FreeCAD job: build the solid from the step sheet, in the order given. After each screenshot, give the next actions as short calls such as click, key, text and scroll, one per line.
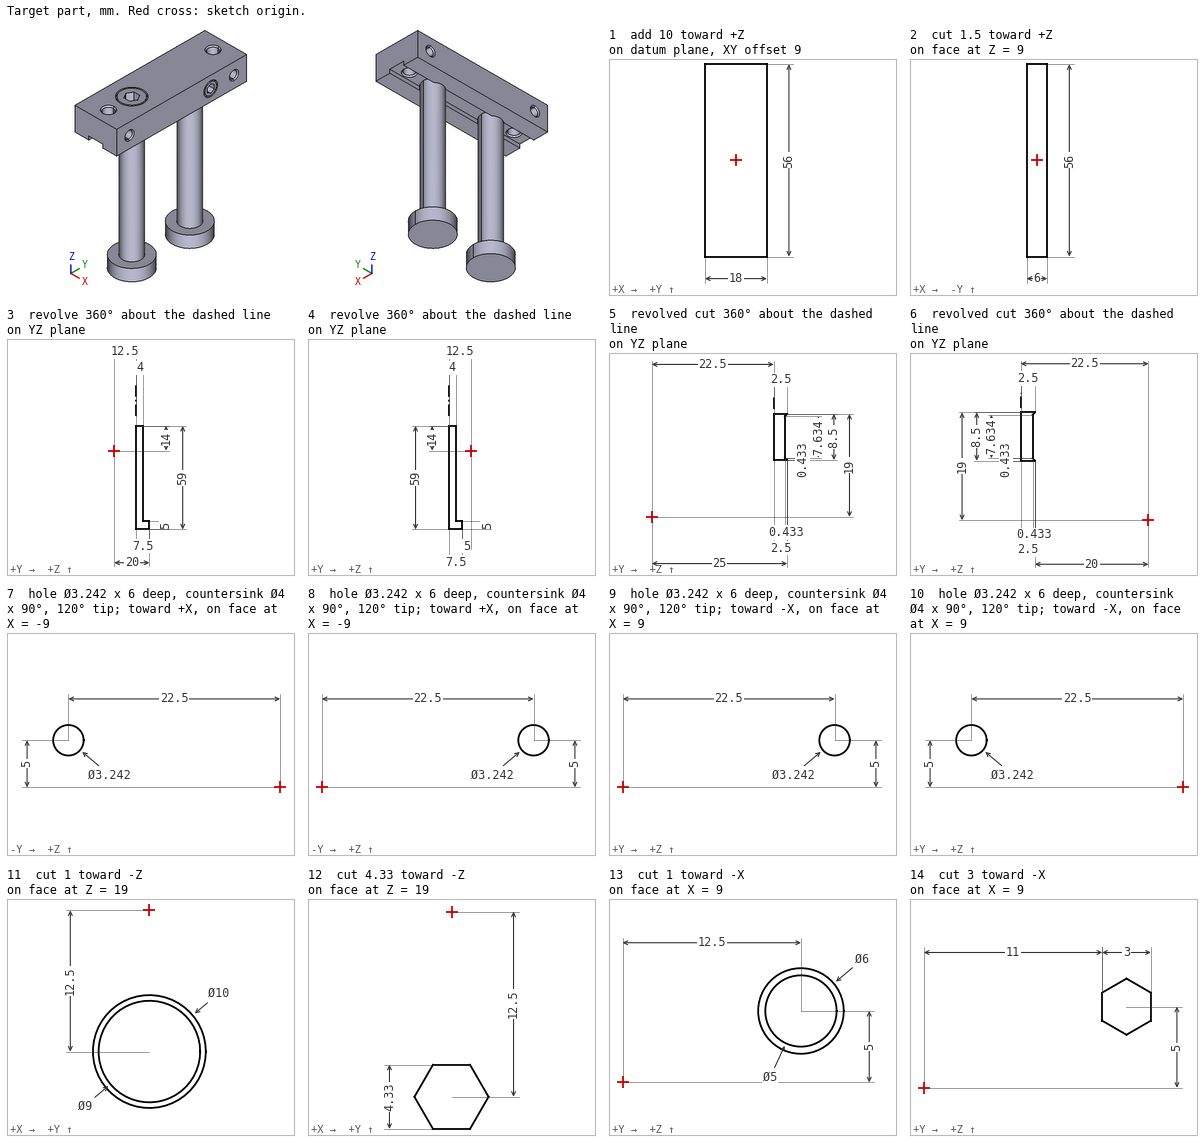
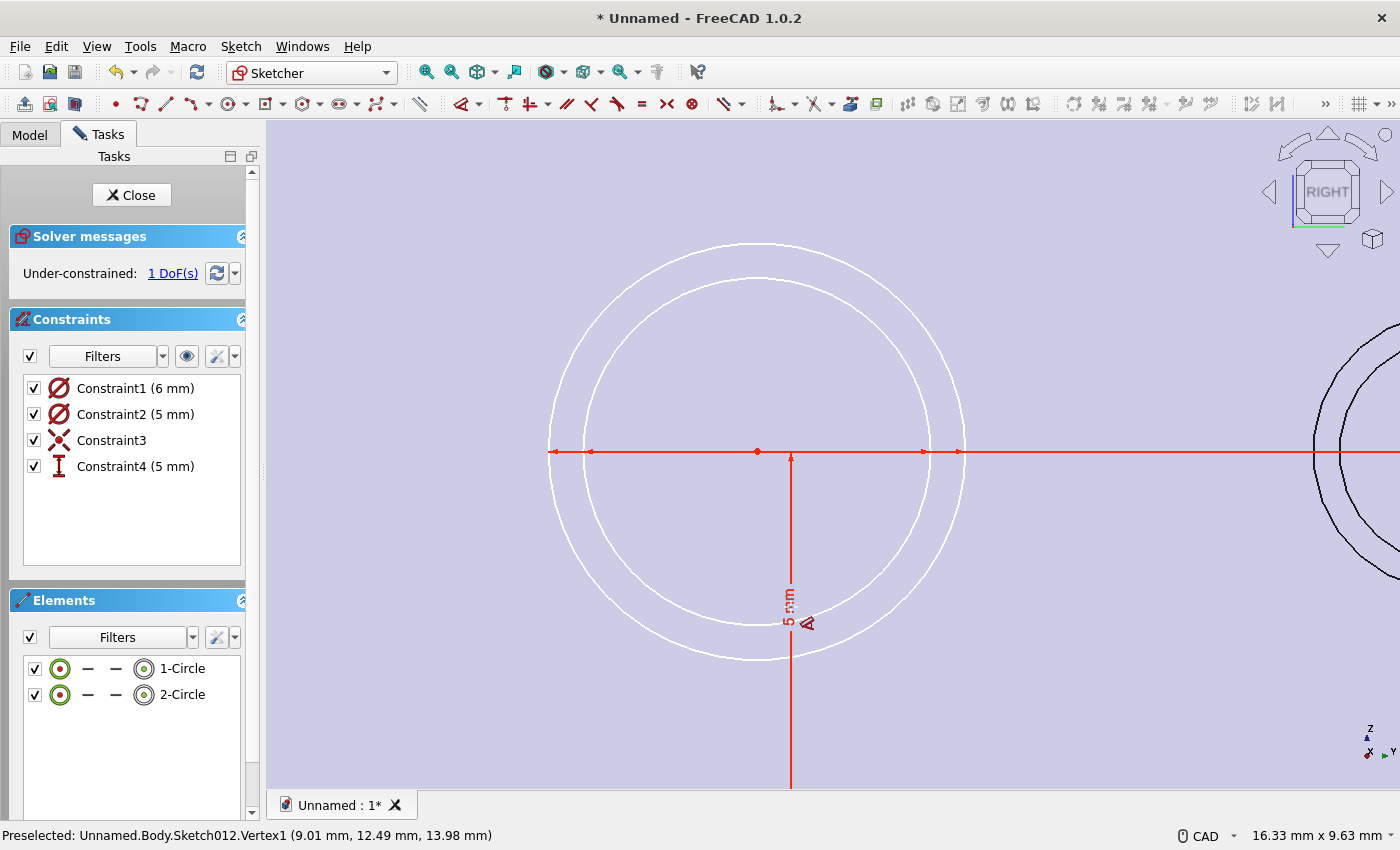
click(757, 452)
click(525, 418)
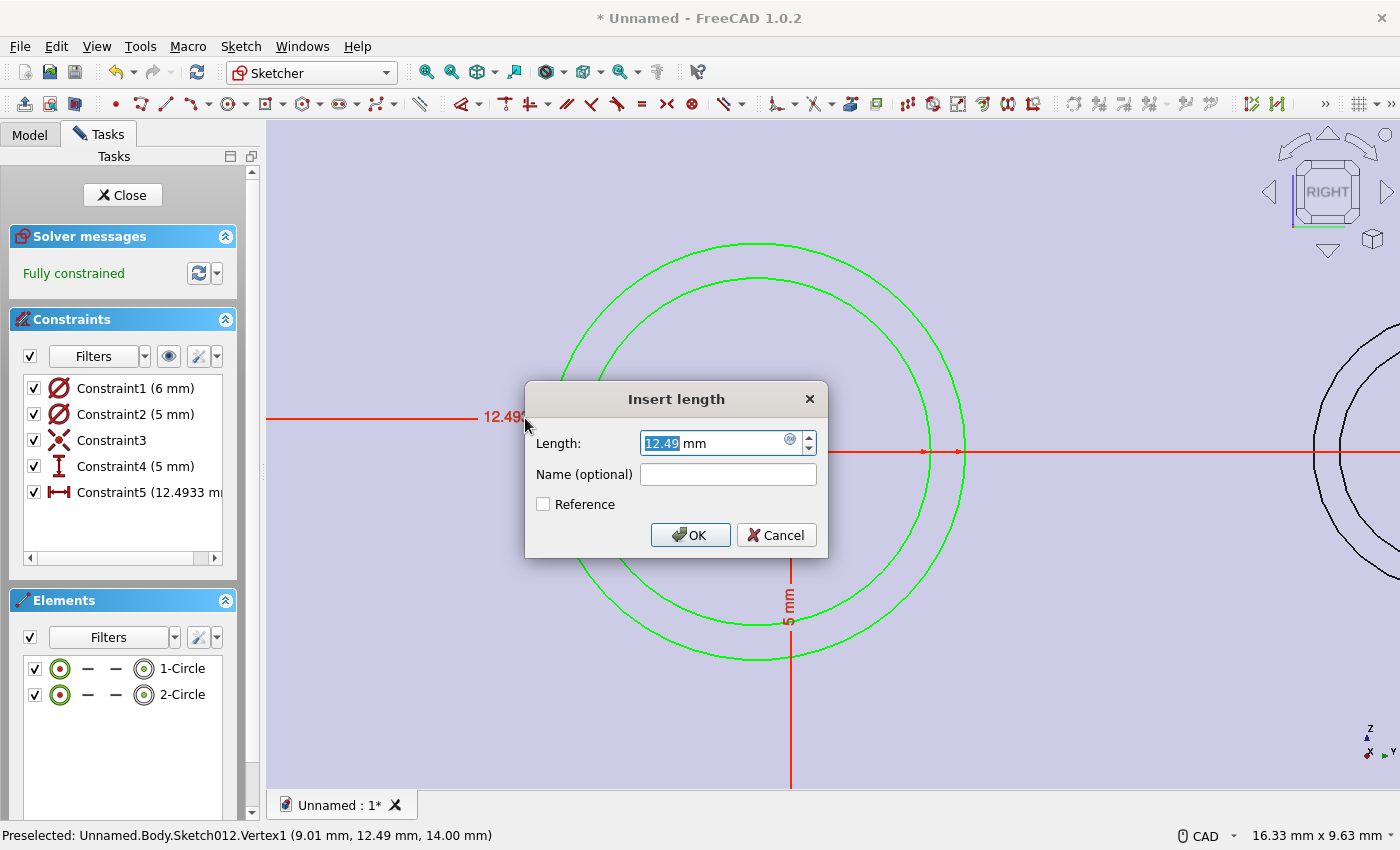
text(12.5)
key(Return)
key(Escape)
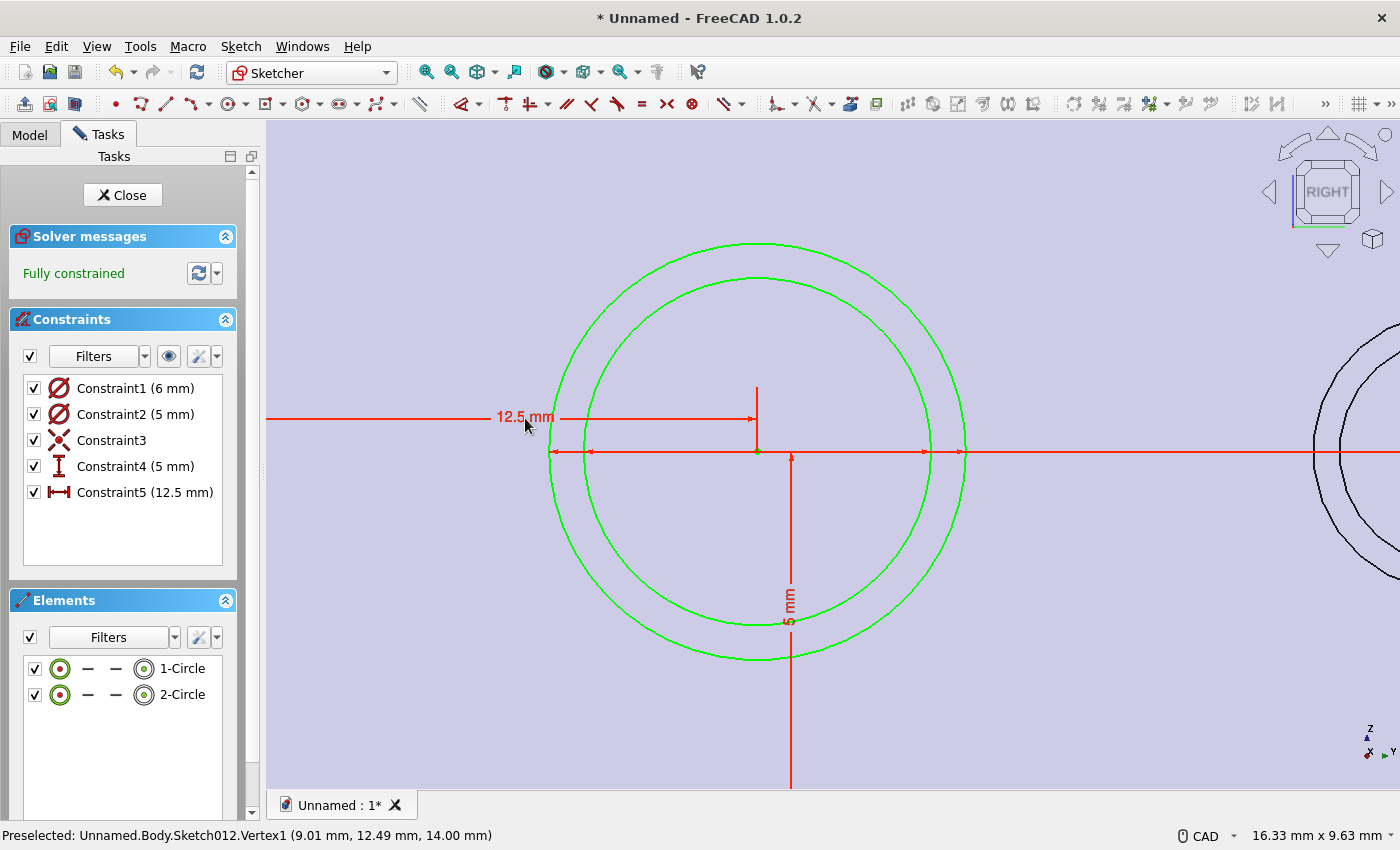
click(123, 195)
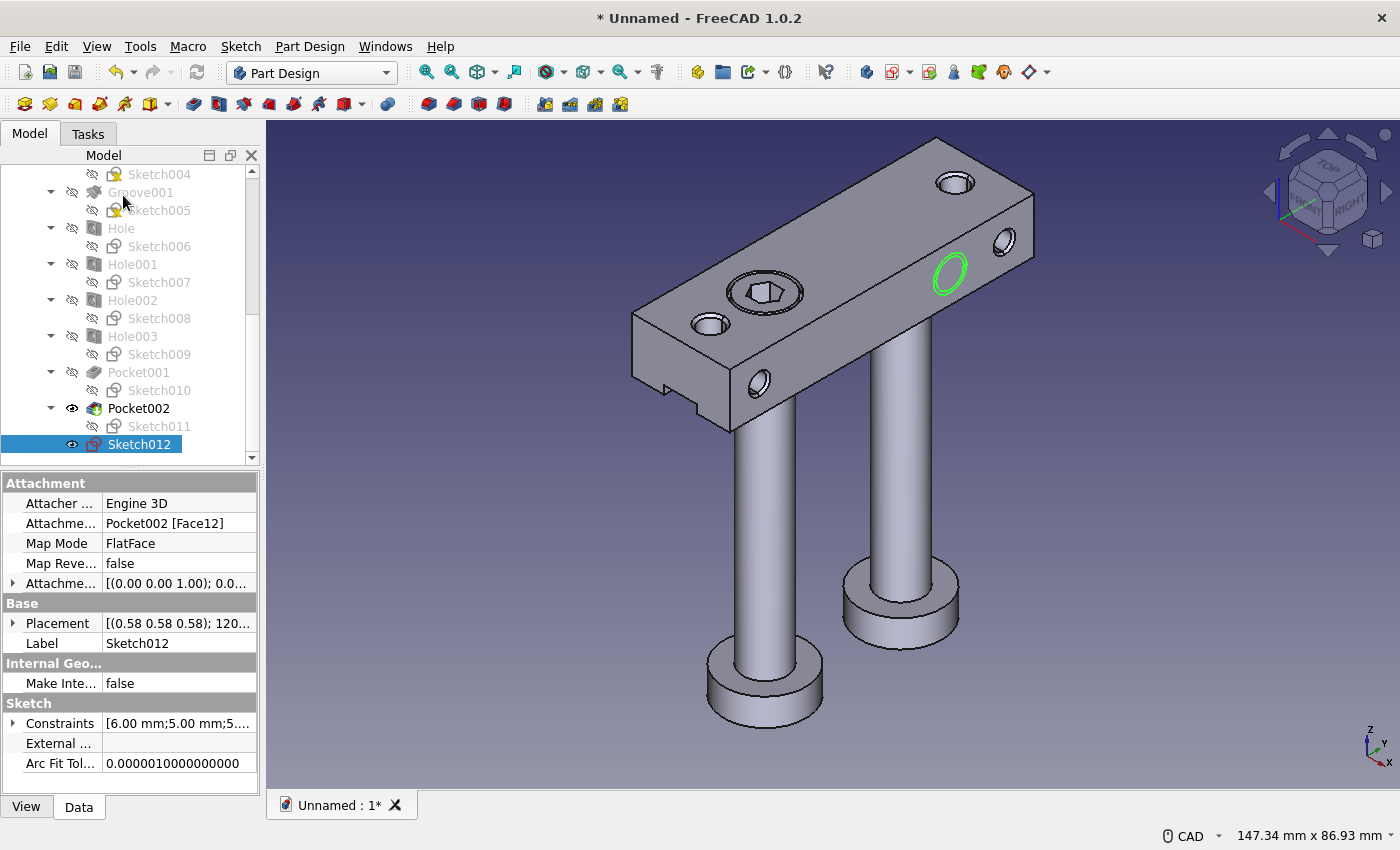
click(194, 104)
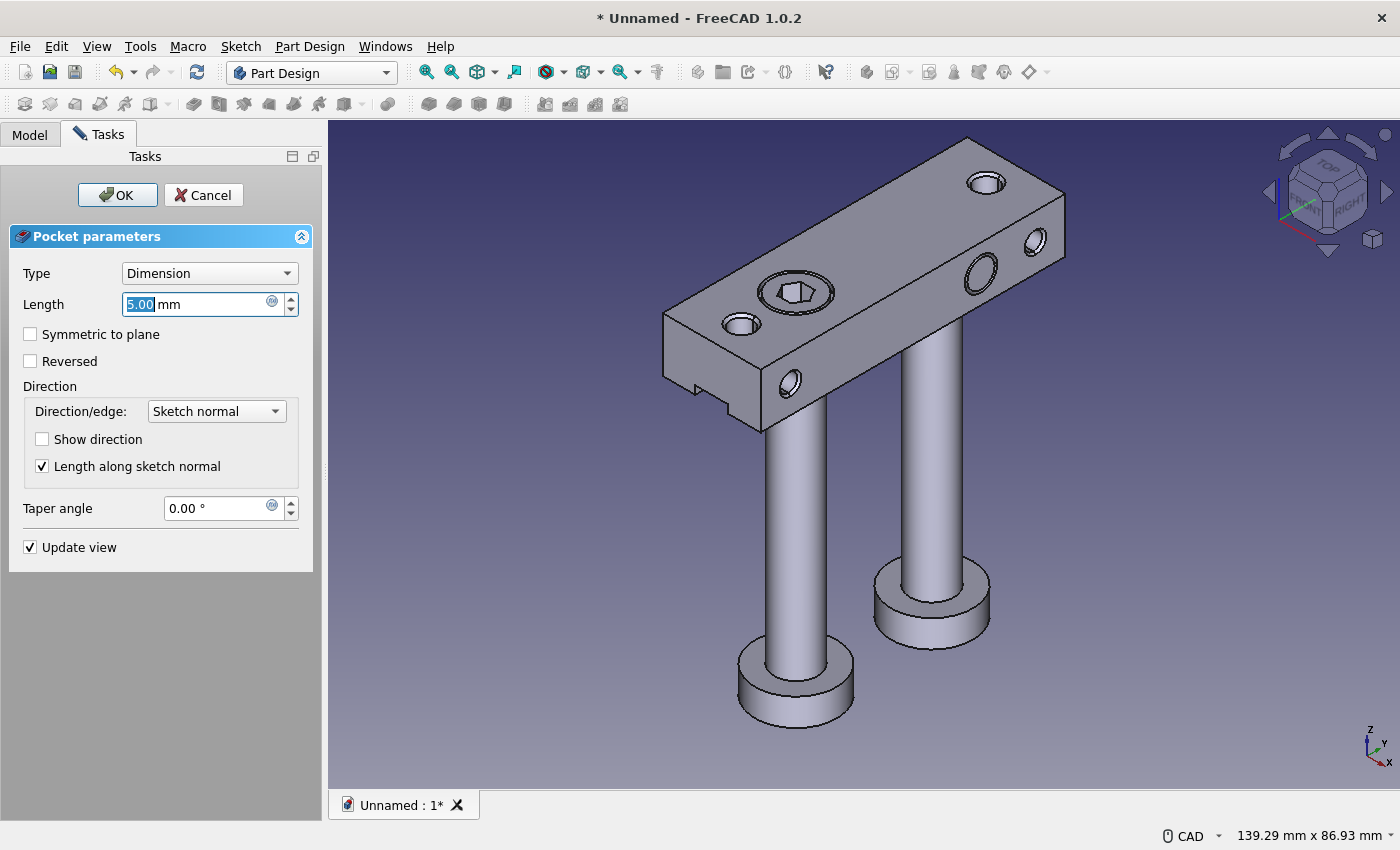
text(1)
key(Tab)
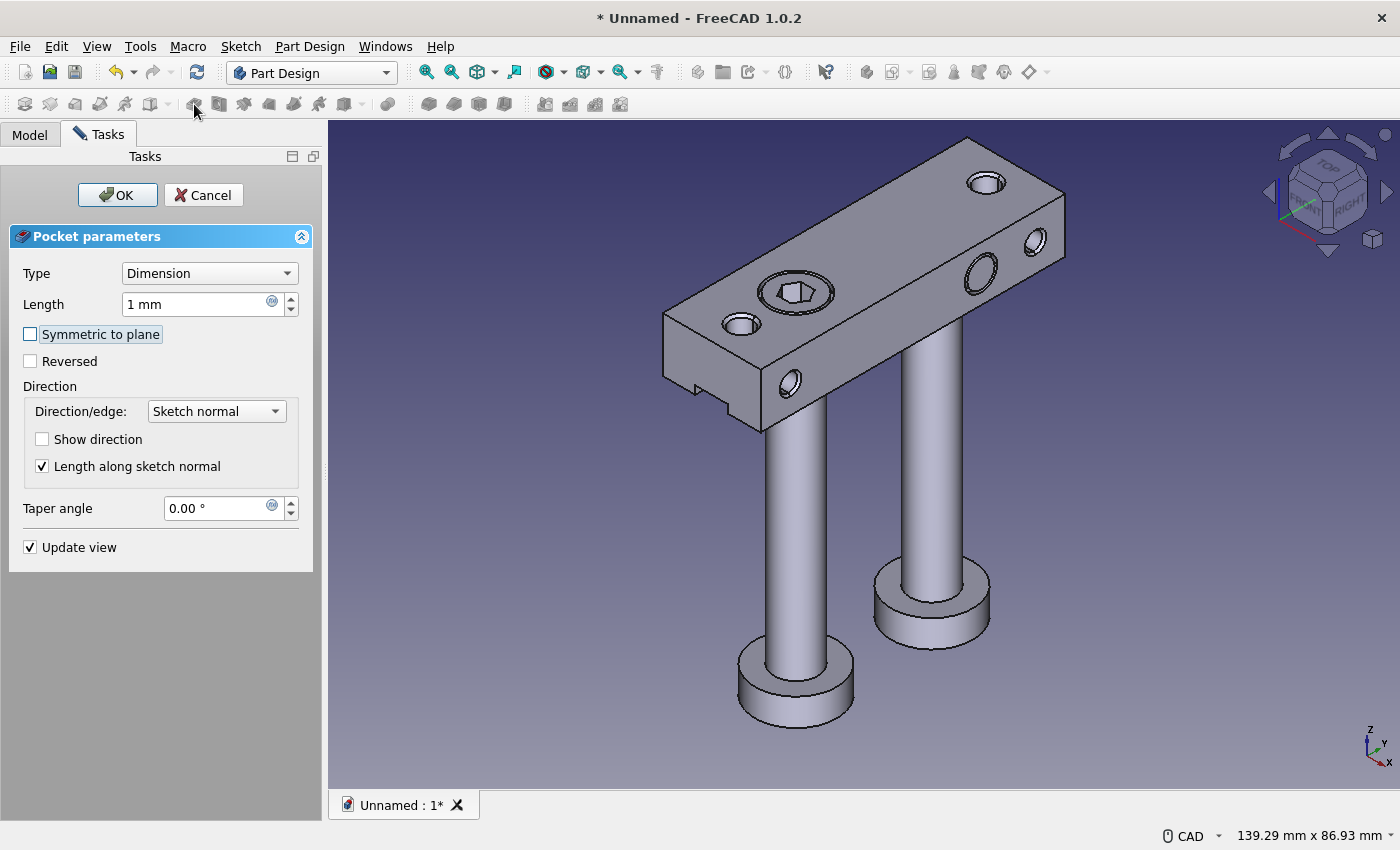
click(118, 195)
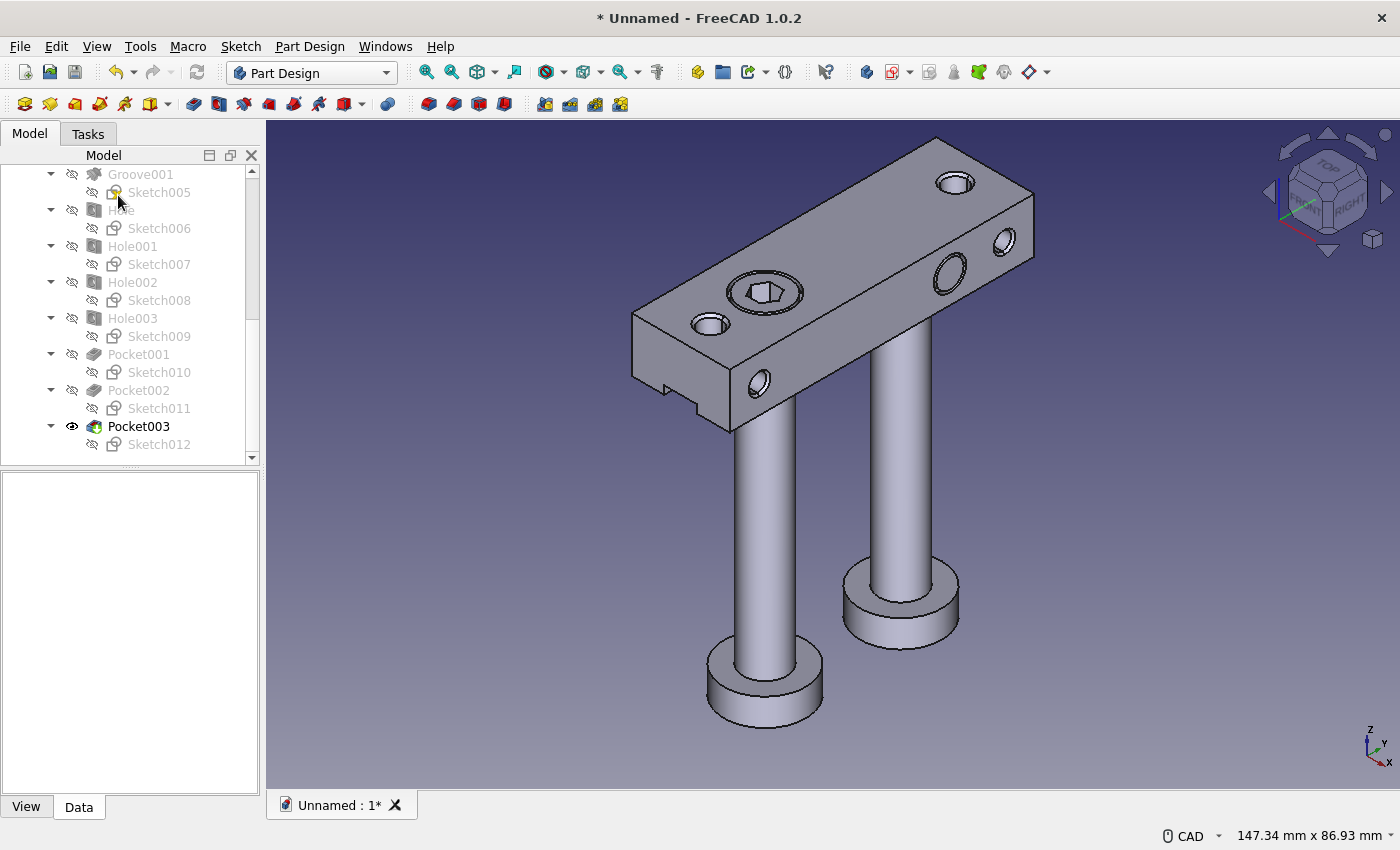
click(882, 312)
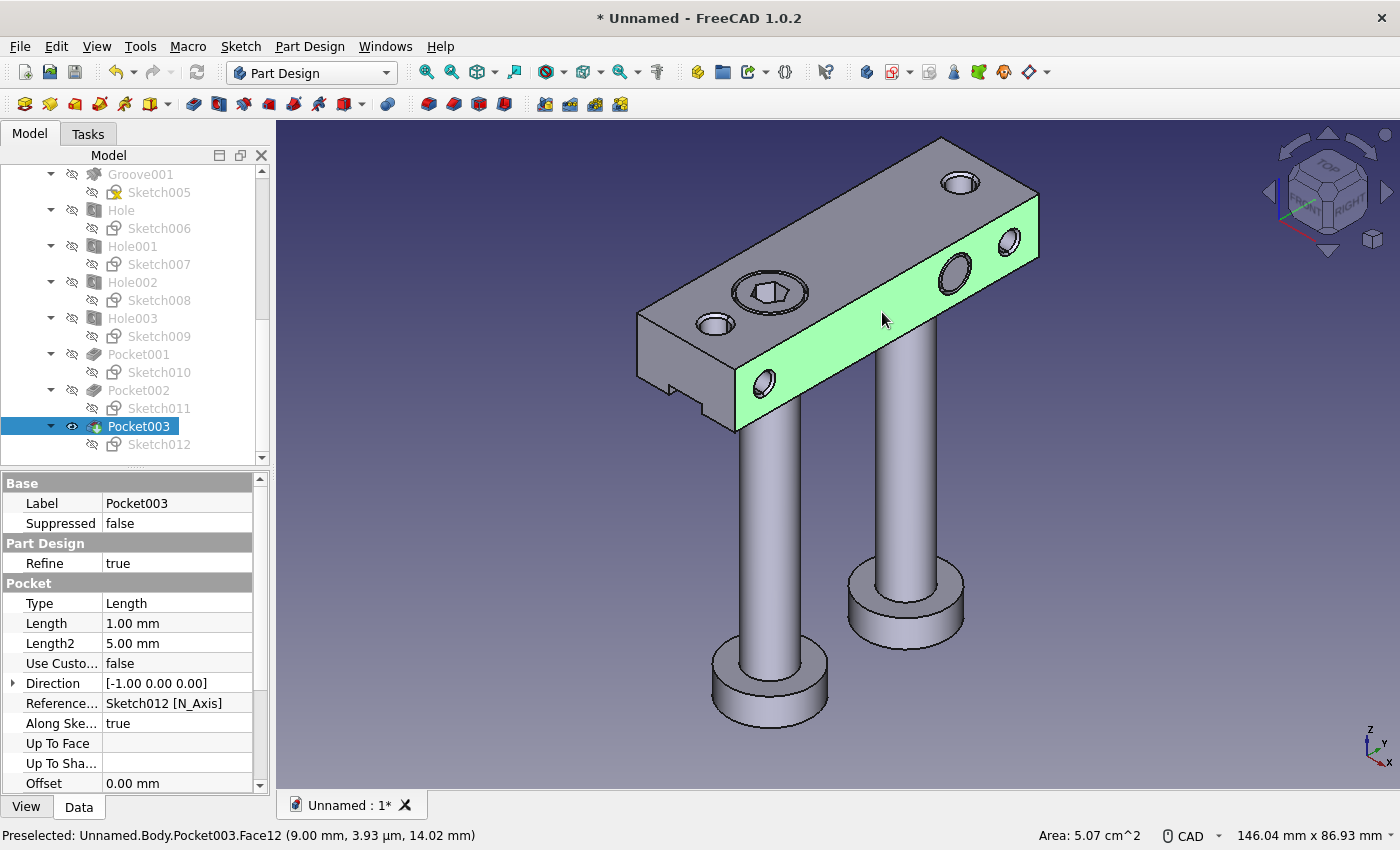
click(892, 72)